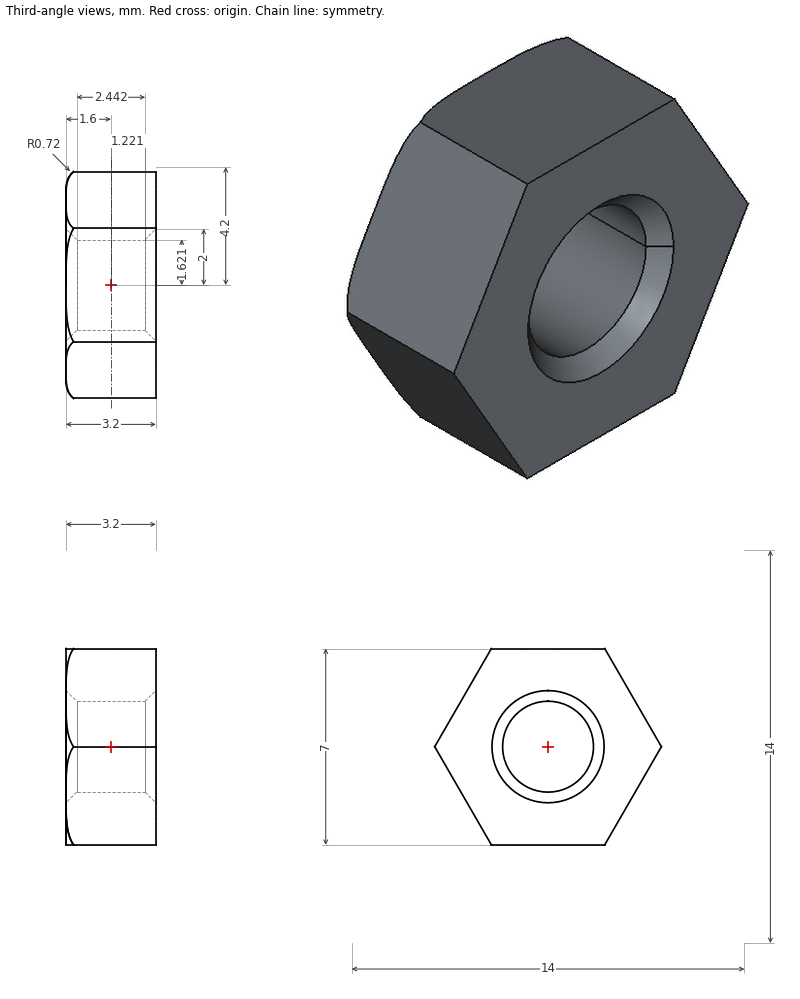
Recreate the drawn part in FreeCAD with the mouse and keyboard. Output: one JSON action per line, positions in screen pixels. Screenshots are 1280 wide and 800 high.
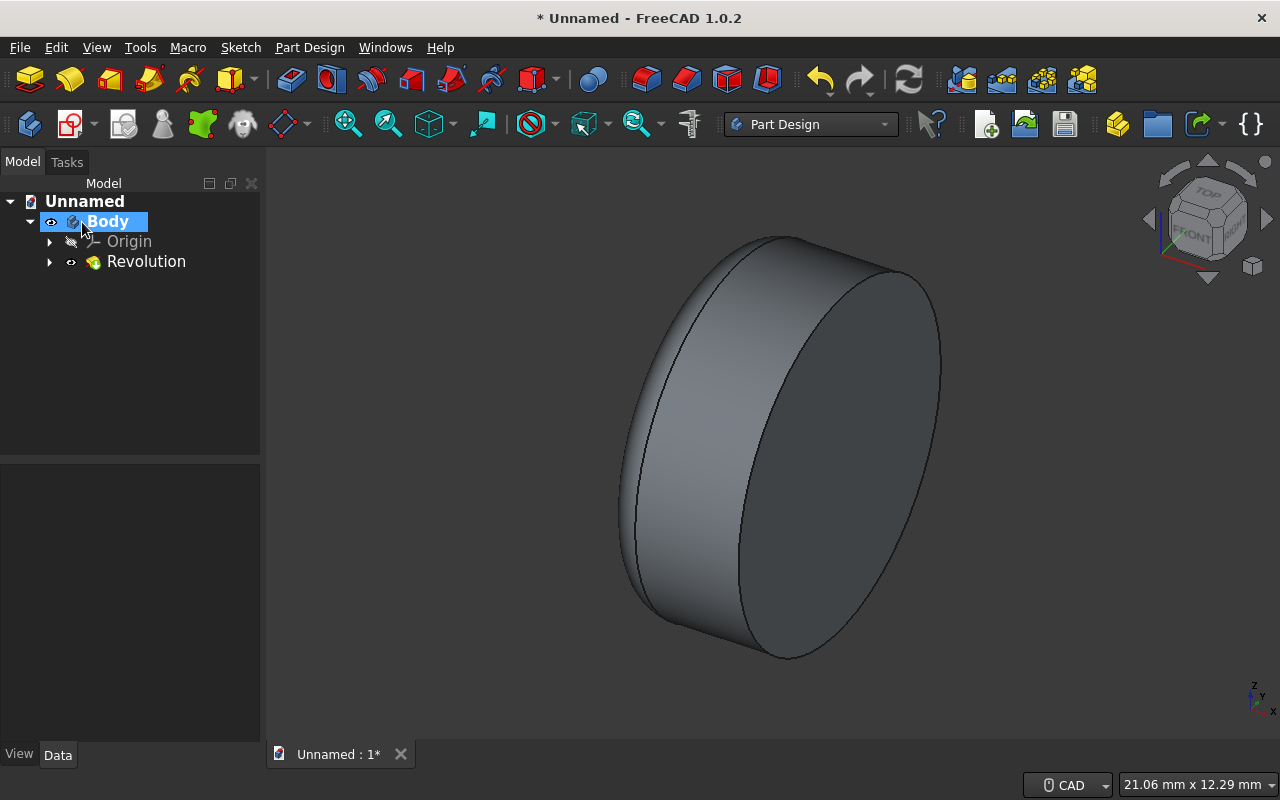
{"action": "left_click", "coordinate": [70, 124]}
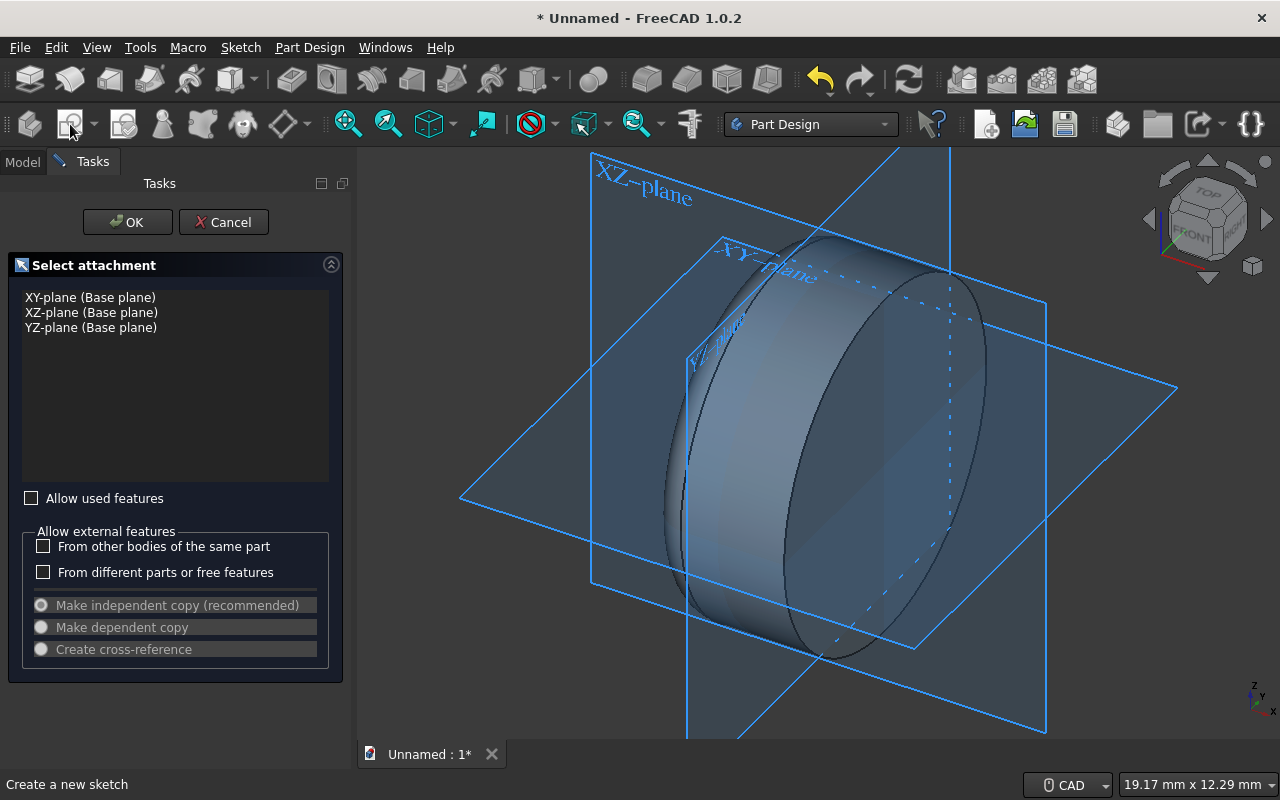
{"action": "left_click", "coordinate": [82, 298]}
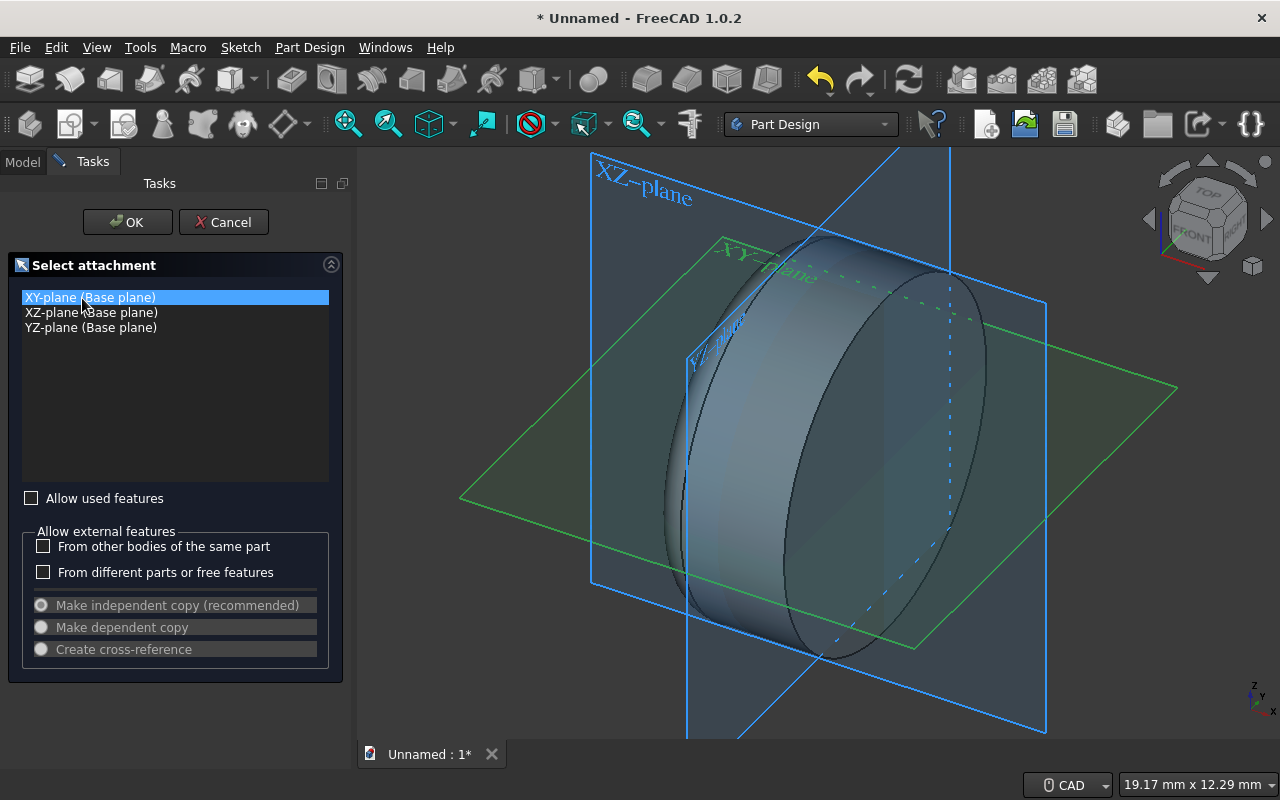
{"action": "left_click", "coordinate": [128, 222]}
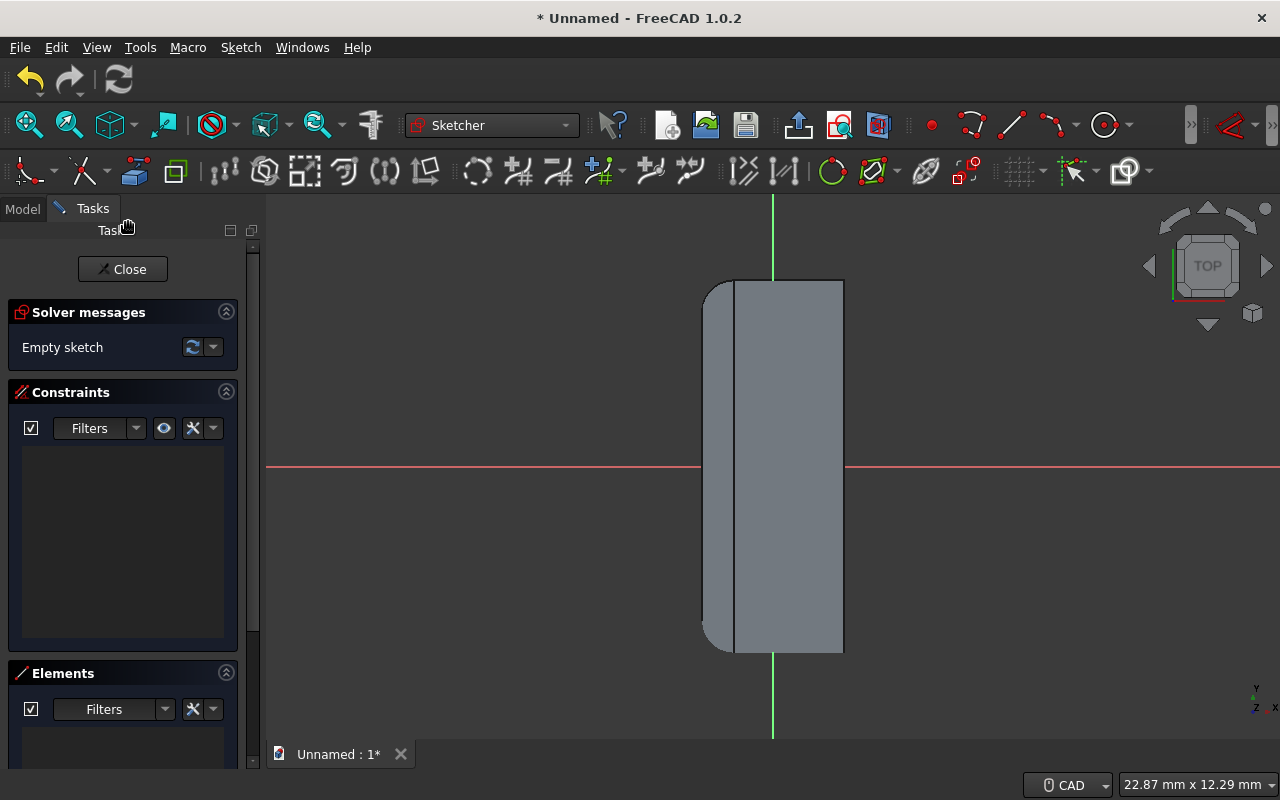
{"action": "key", "text": "q s"}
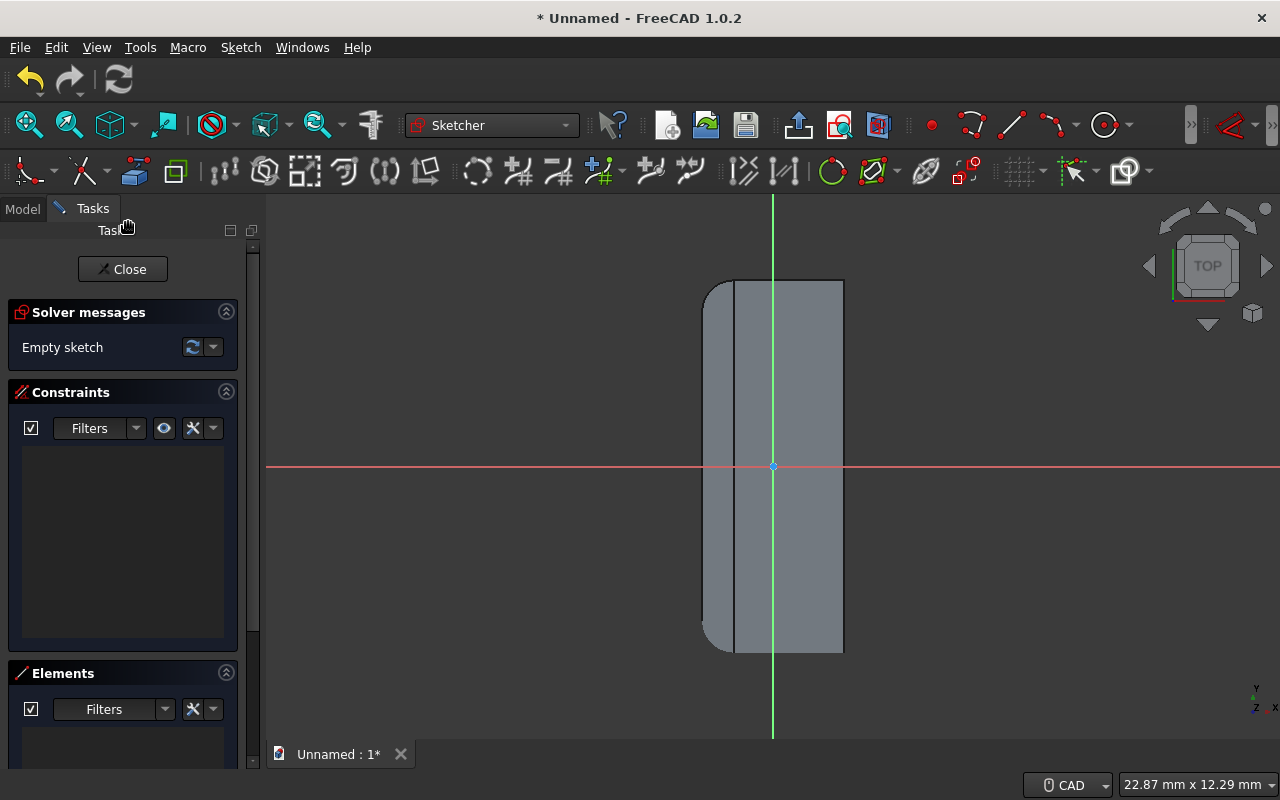
{"action": "scroll", "coordinate": [795, 408], "scroll_direction": "up", "scroll_amount": 7}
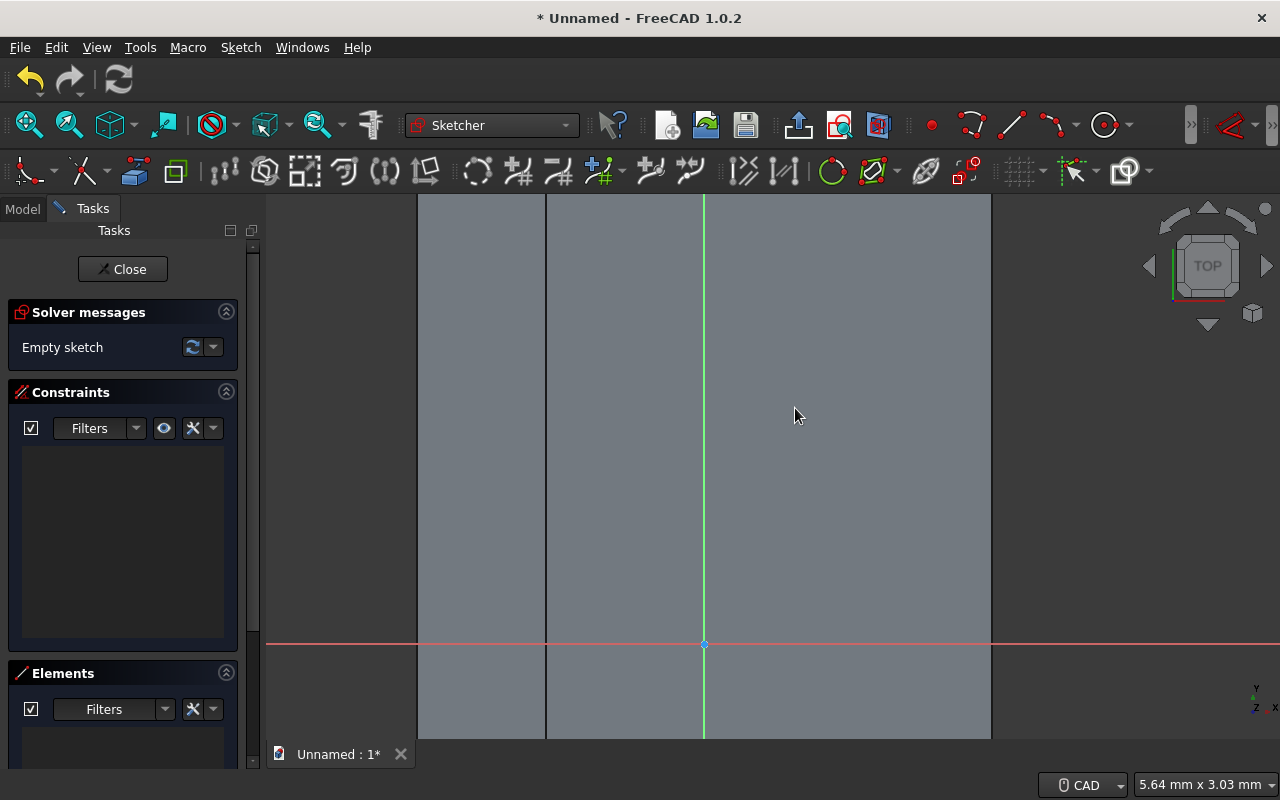
{"action": "key", "text": "g m"}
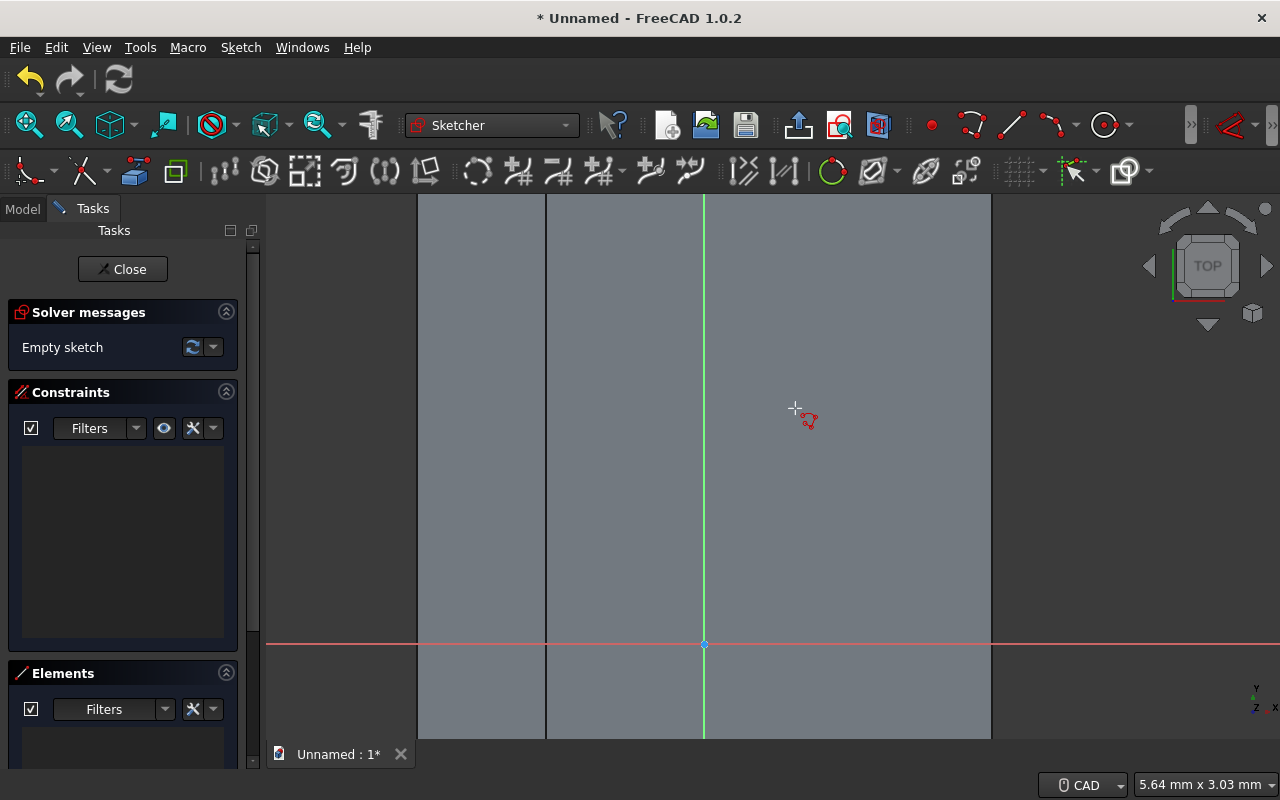
{"action": "left_click", "coordinate": [417, 644]}
{"action": "left_click", "coordinate": [992, 635]}
{"action": "left_click", "coordinate": [992, 284]}
{"action": "left_click", "coordinate": [924, 353]}
{"action": "left_click", "coordinate": [485, 353]}
{"action": "left_click", "coordinate": [417, 284]}
{"action": "left_click", "coordinate": [417, 644]}
{"action": "key", "text": "Escape"}
{"action": "key", "text": "Escape"}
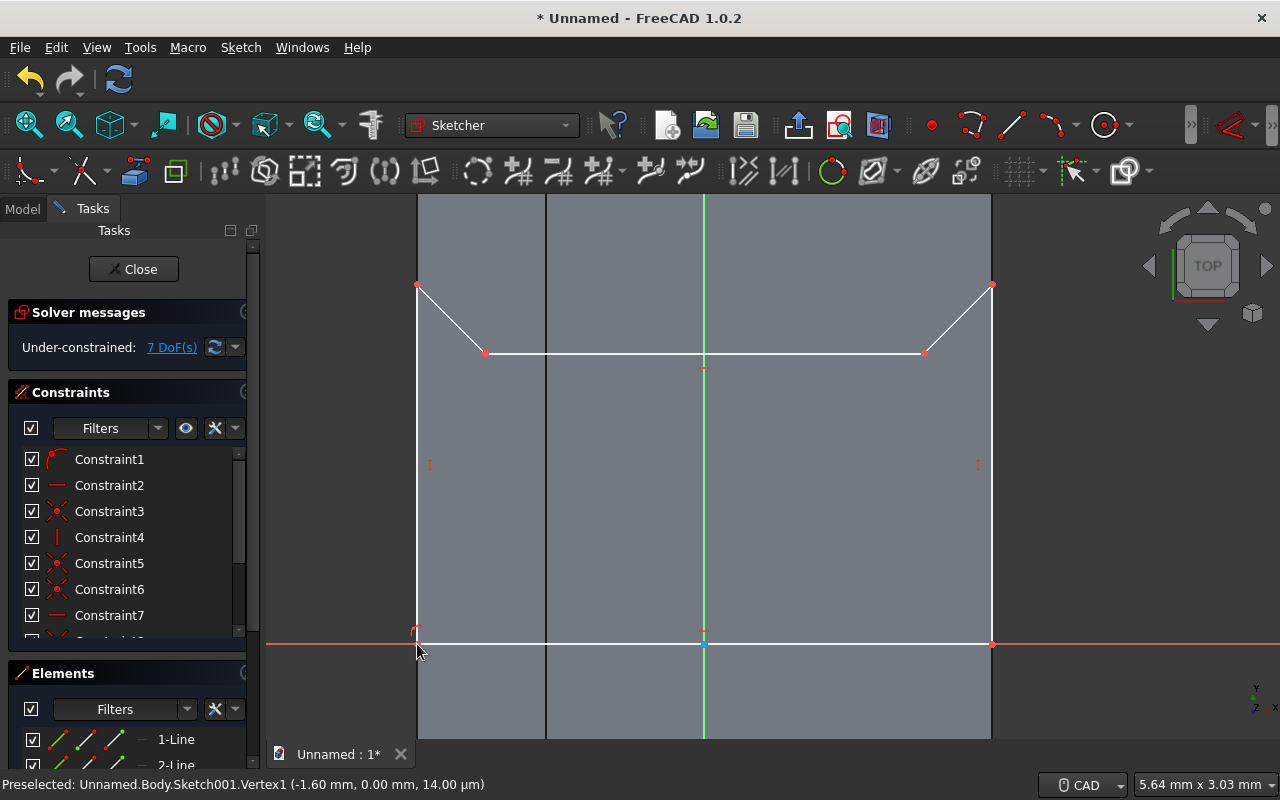
{"action": "left_click", "coordinate": [992, 285]}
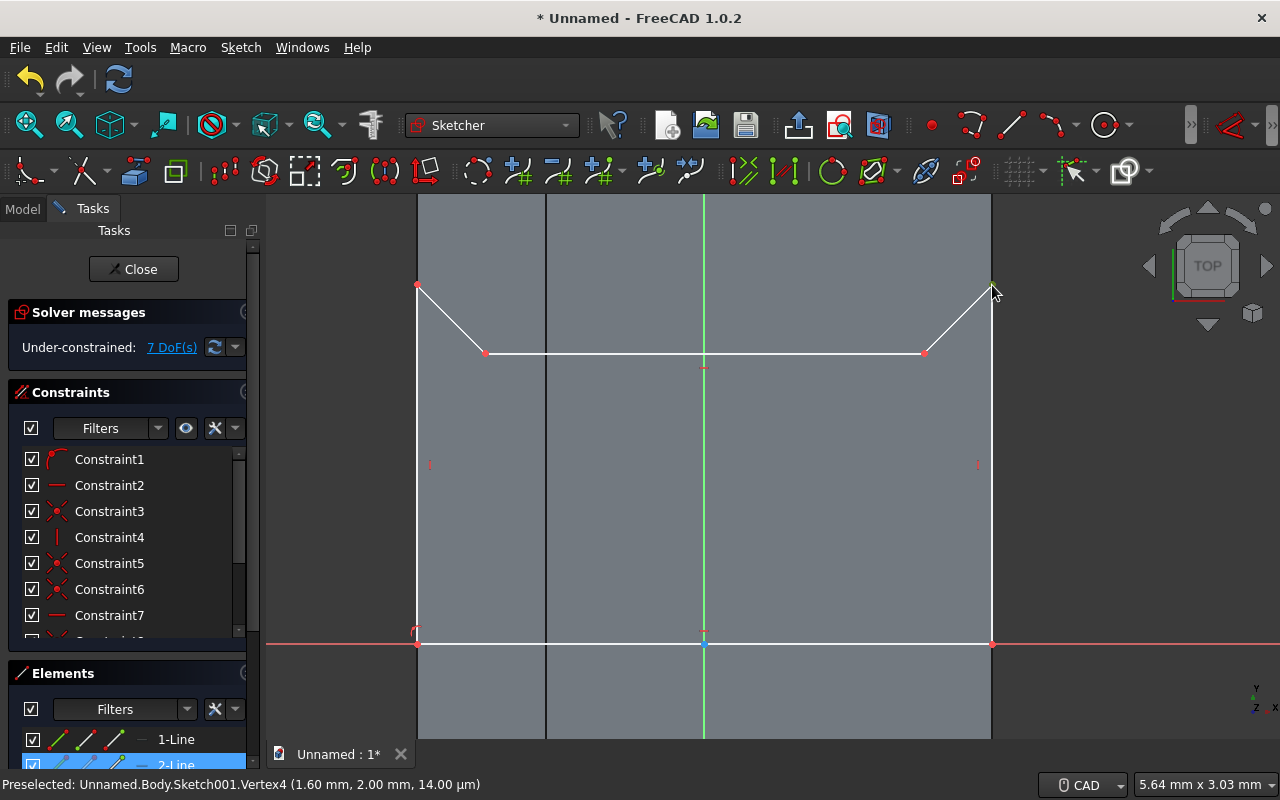
{"action": "left_click", "coordinate": [417, 285]}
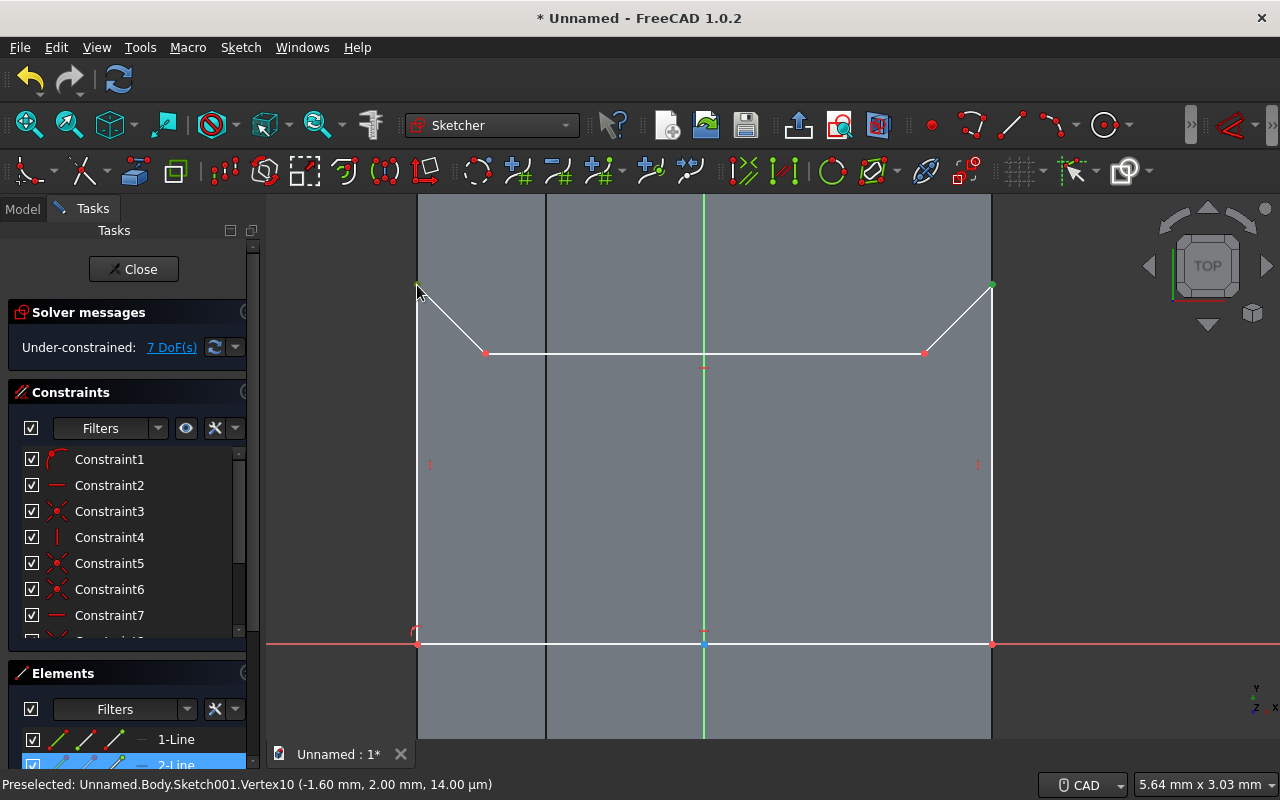
{"action": "left_click", "coordinate": [704, 676]}